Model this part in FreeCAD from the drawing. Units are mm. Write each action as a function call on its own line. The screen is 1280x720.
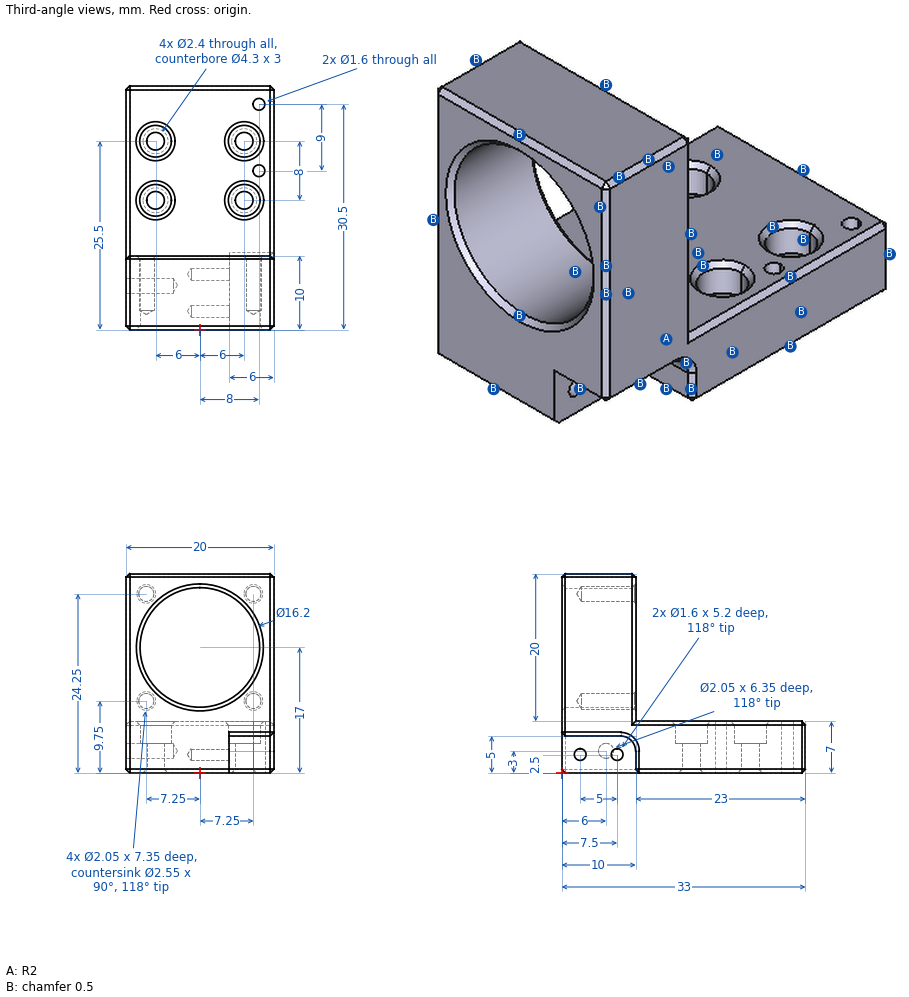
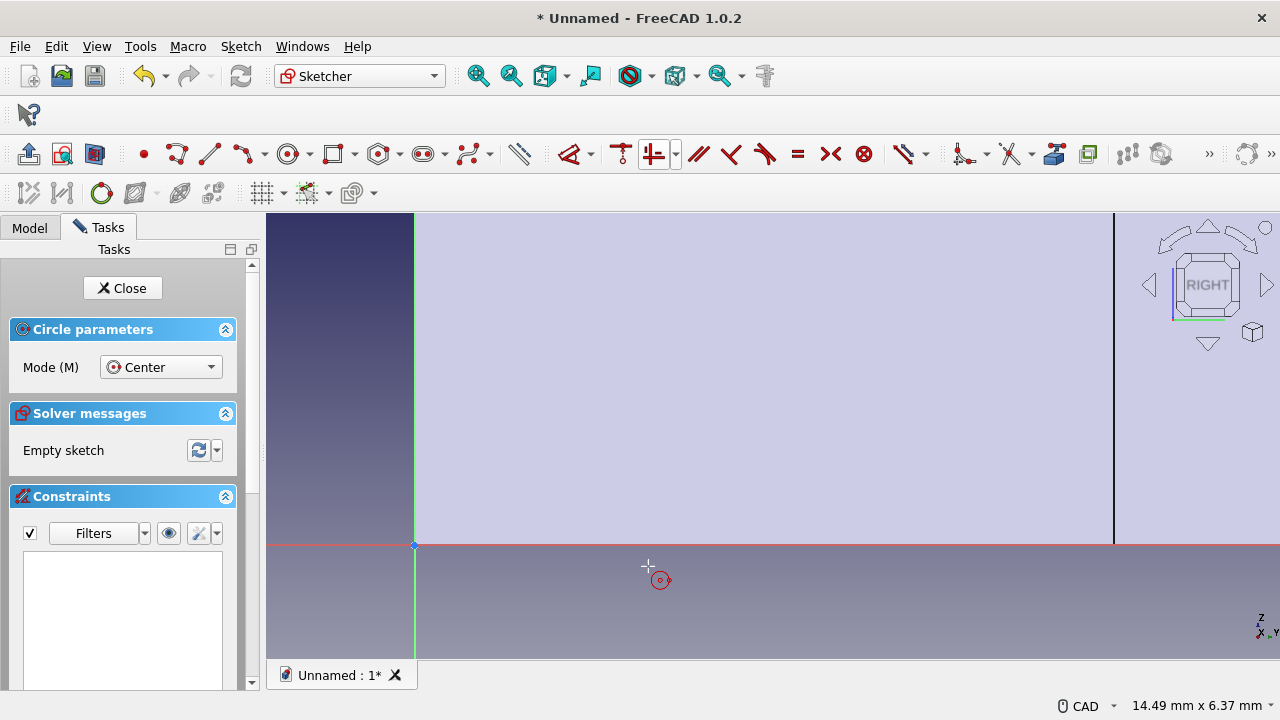
click(939, 370)
move(979, 330)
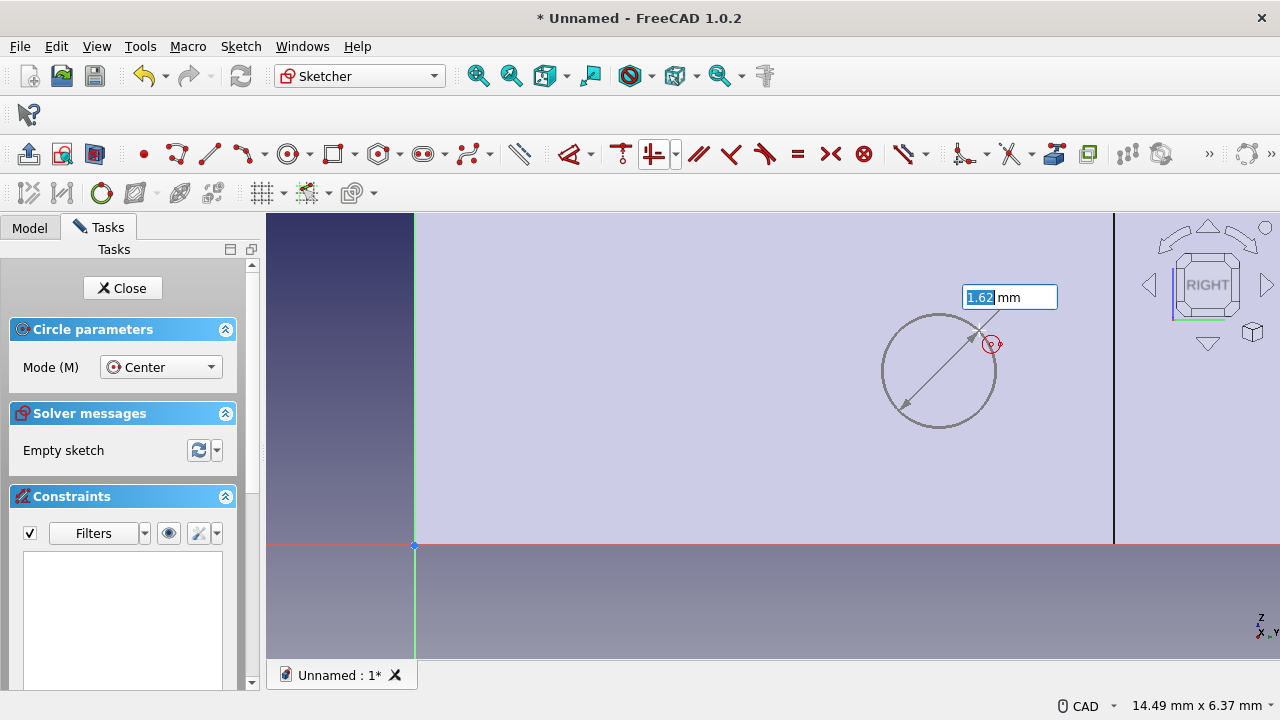
text(1.6)
key(Return)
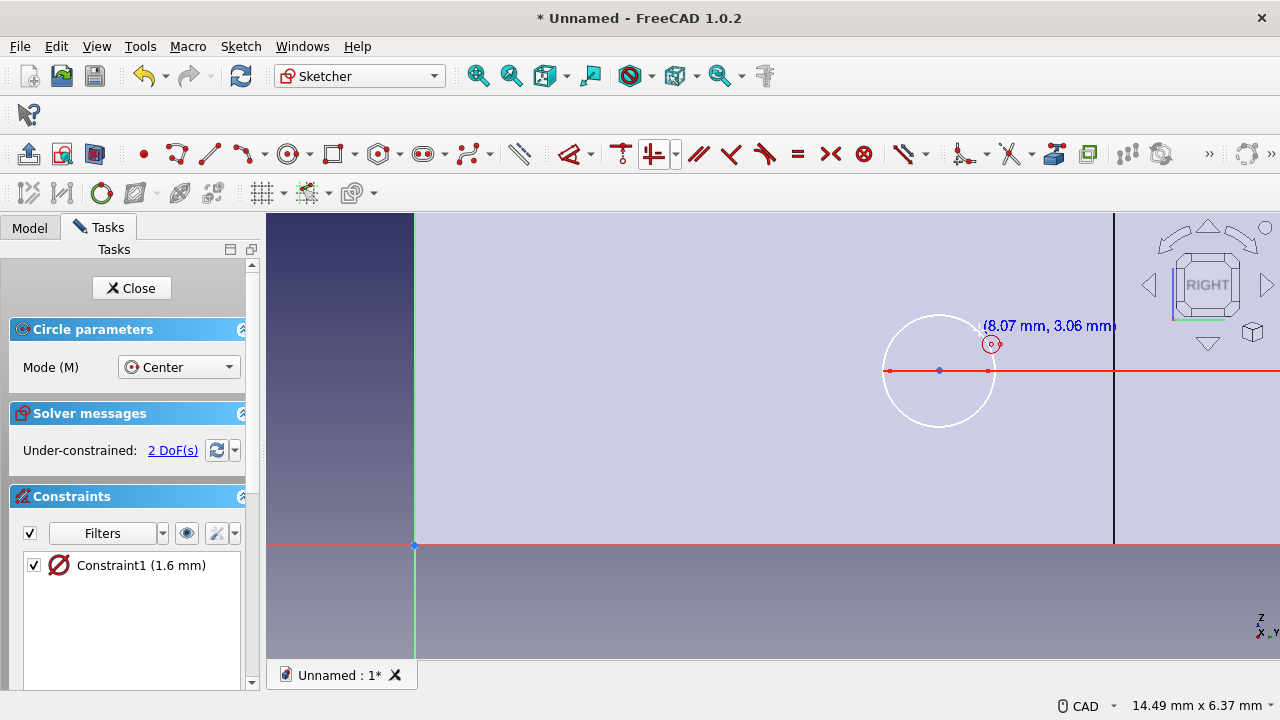
click(590, 370)
move(629, 330)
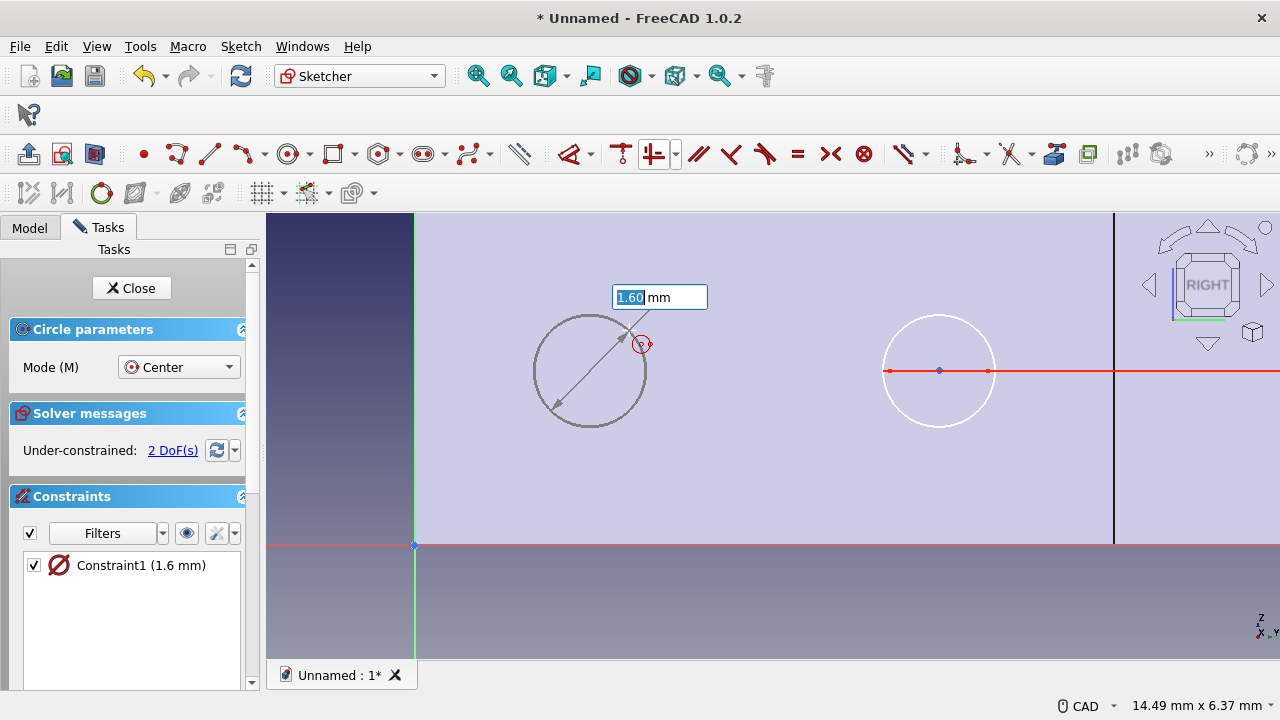
text(1.6)
key(Return)
key(Escape)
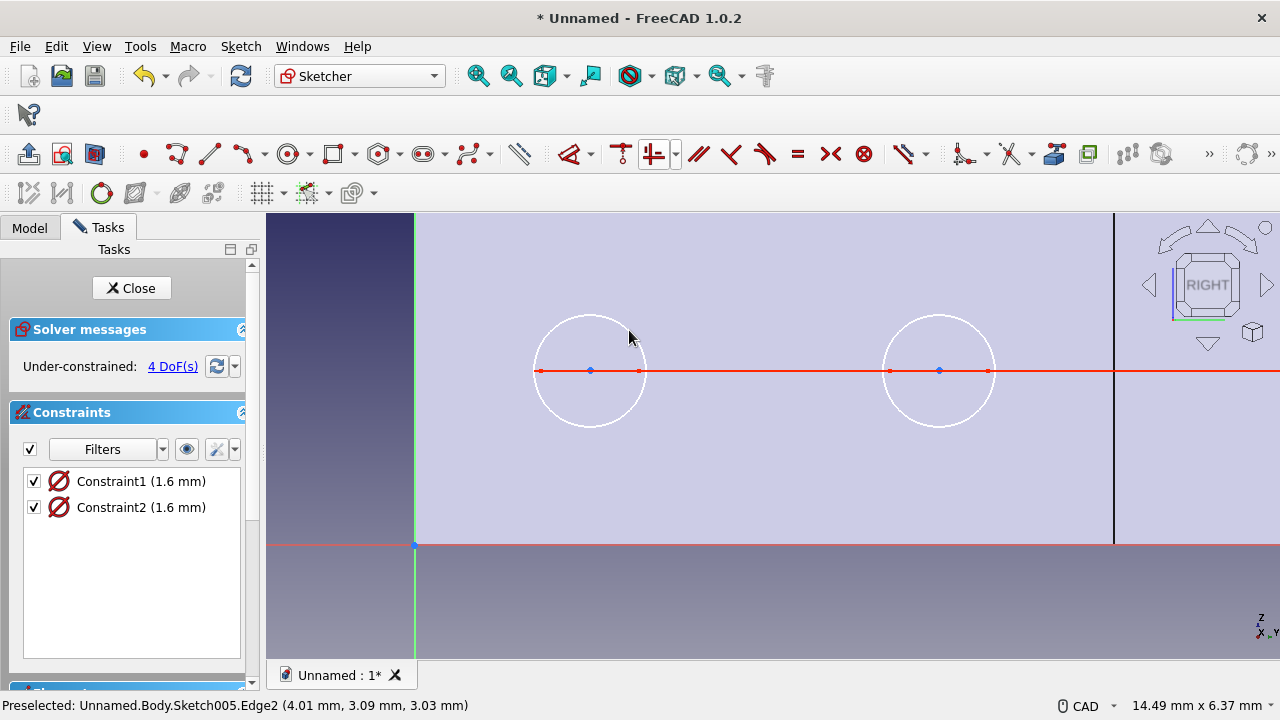
click(939, 371)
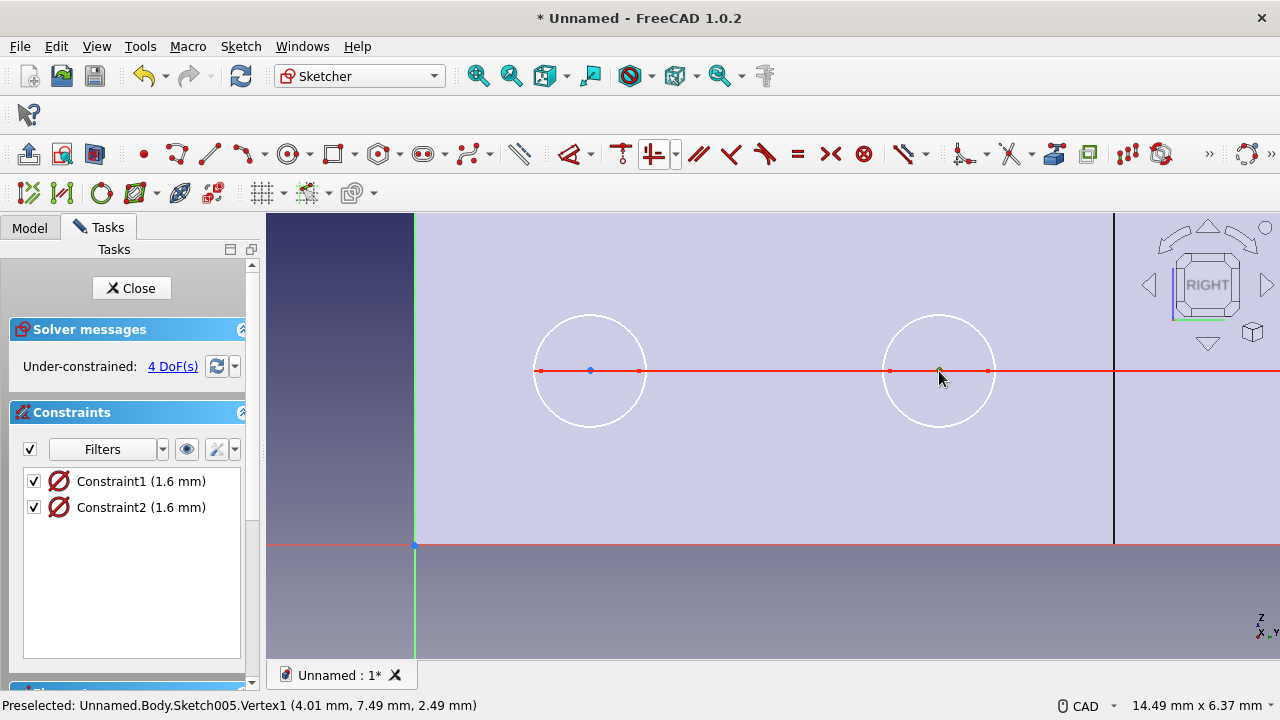
click(590, 371)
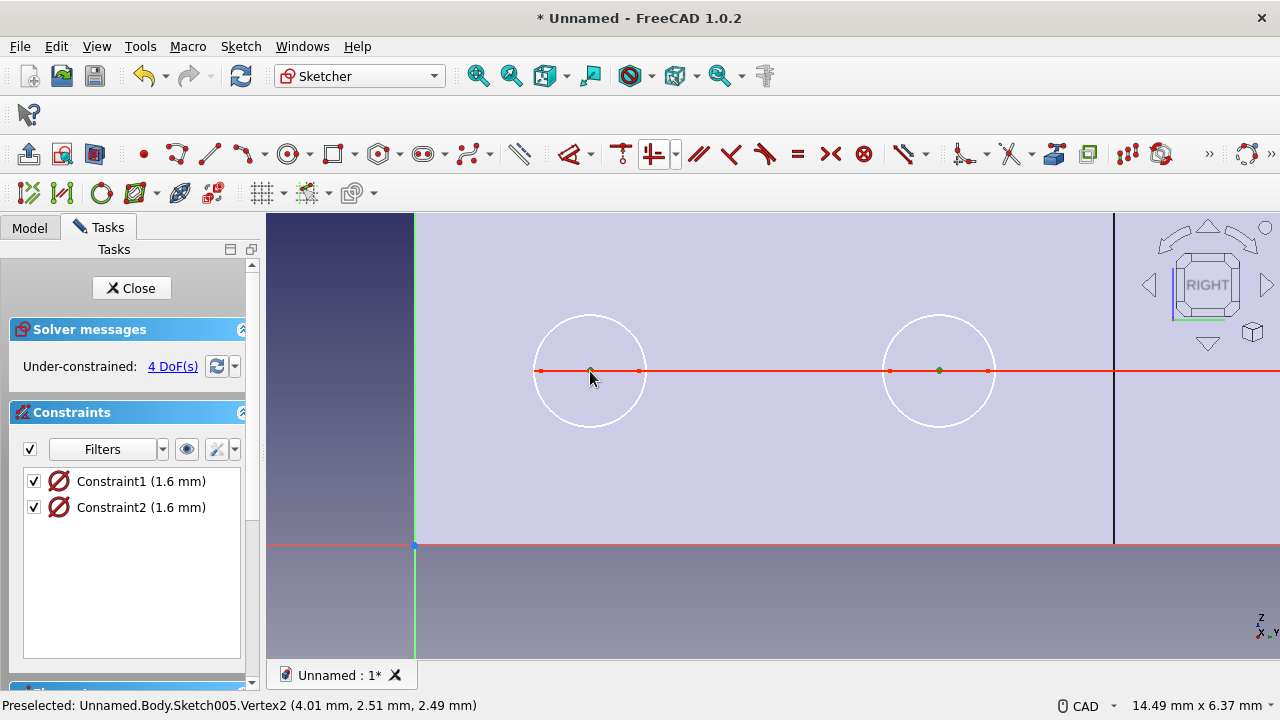
key(h)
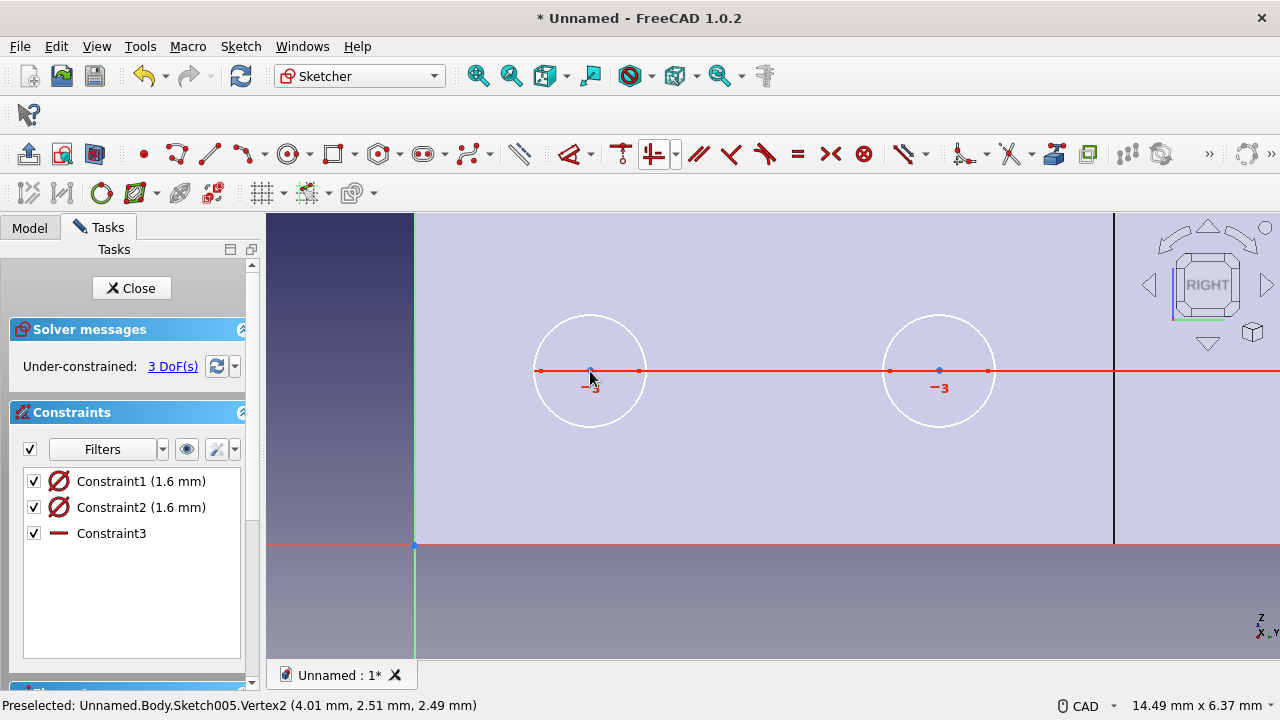
key(d)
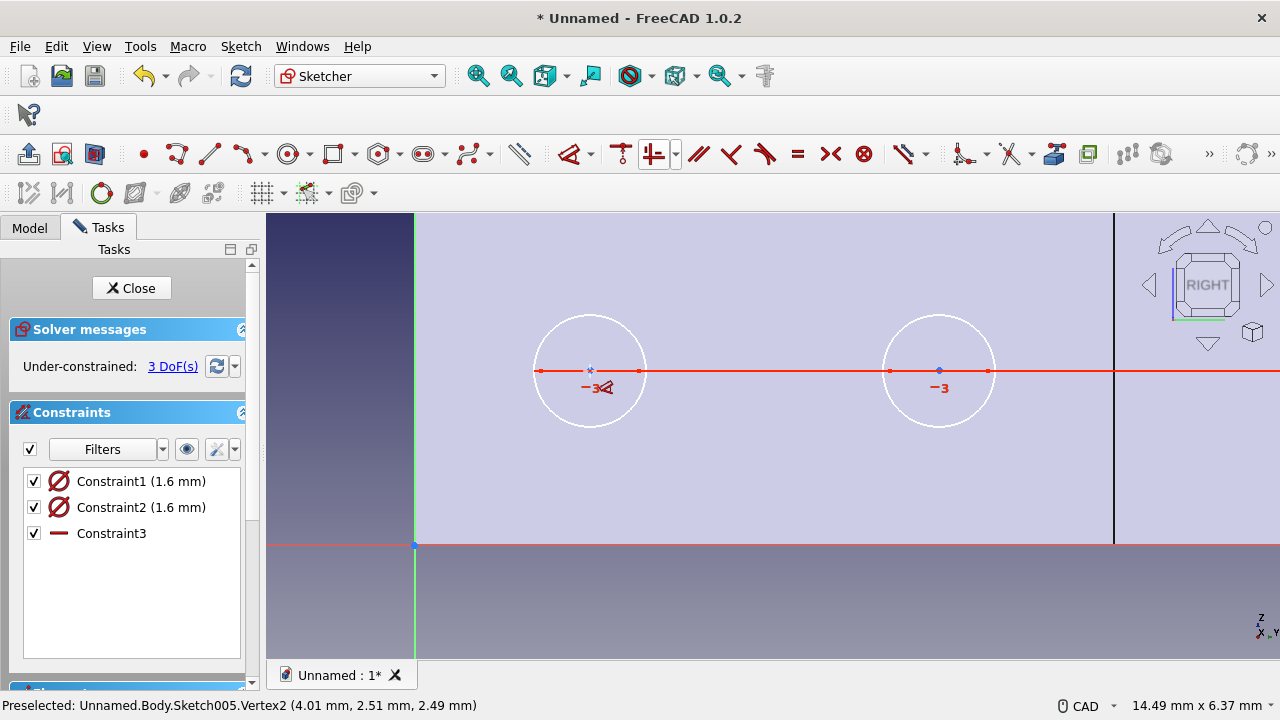
click(939, 371)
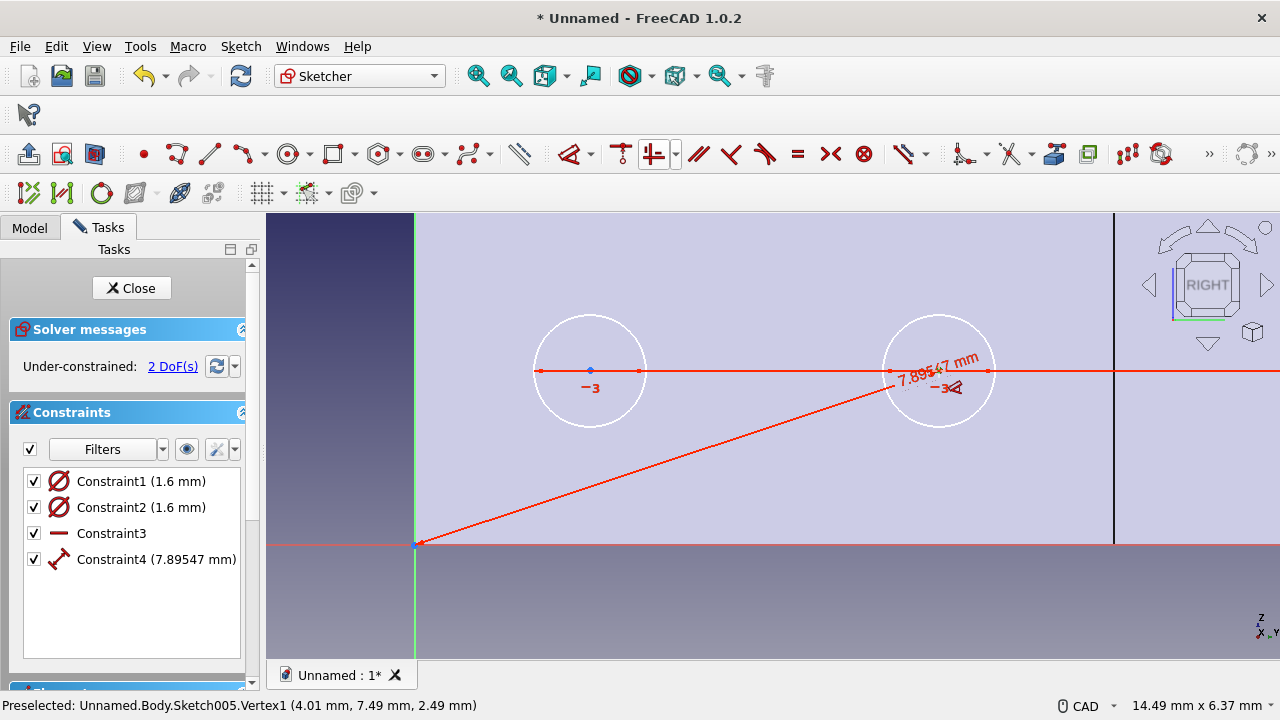
click(590, 371)
click(764, 337)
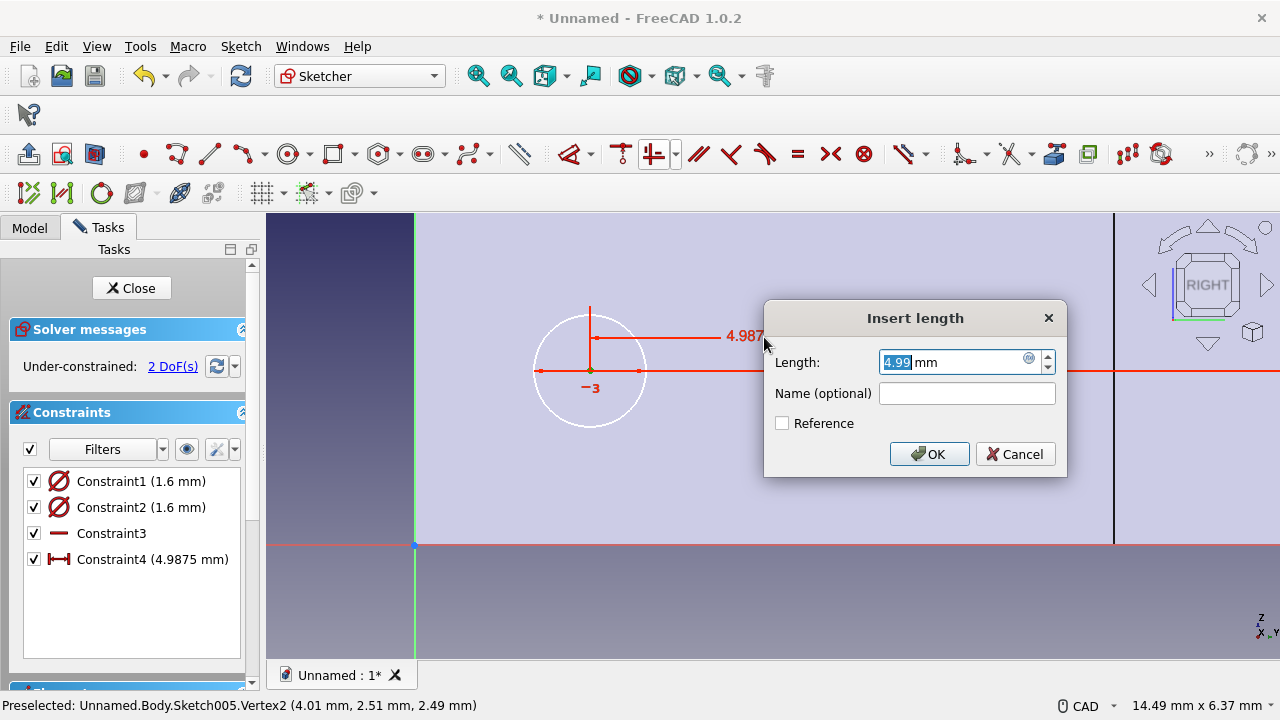
text(5)
key(Return)